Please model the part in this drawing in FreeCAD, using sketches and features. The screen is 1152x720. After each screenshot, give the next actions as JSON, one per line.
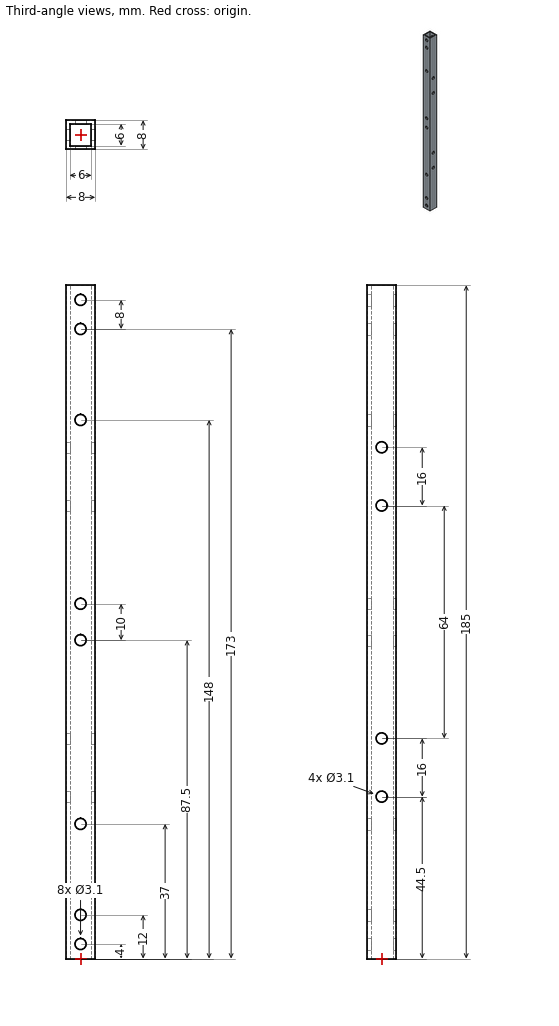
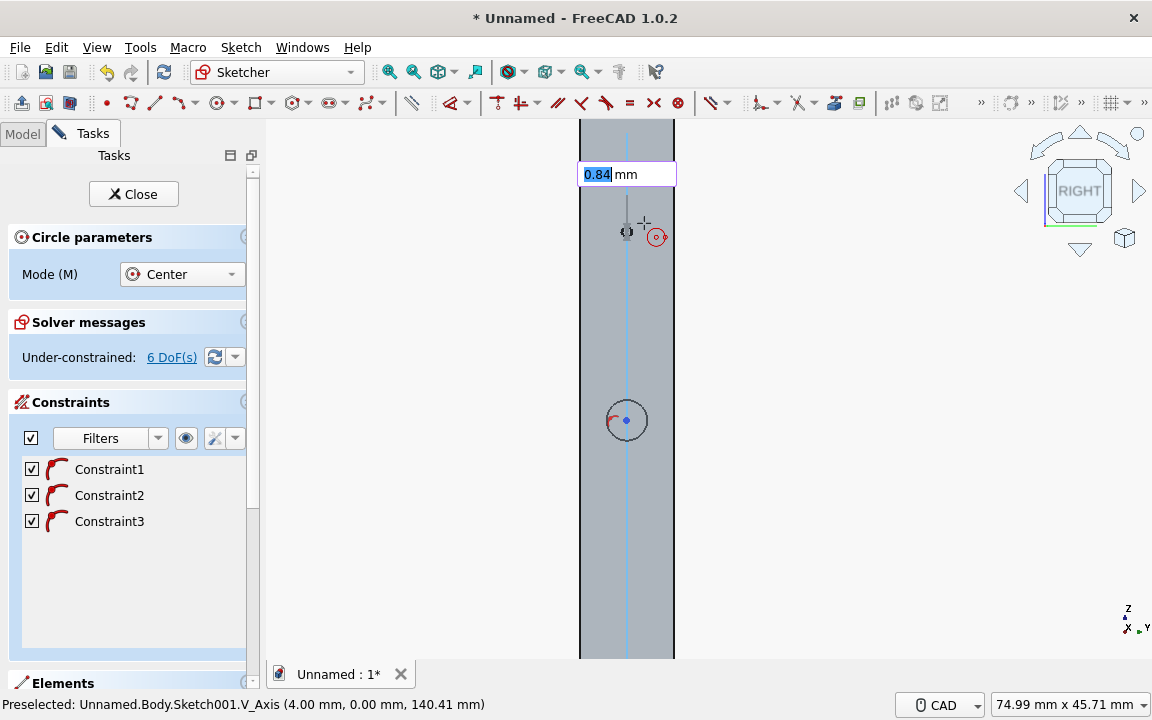
{"action": "left_click", "coordinate": [644, 220]}
{"action": "key", "text": "Escape"}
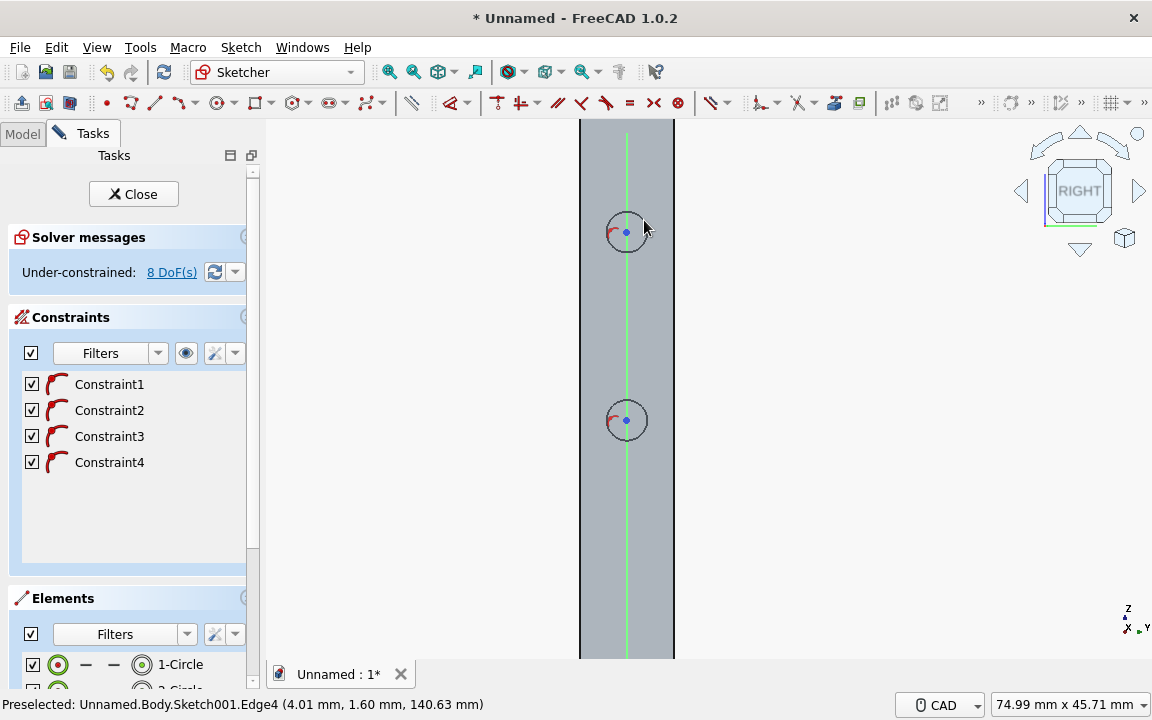
{"action": "scroll", "coordinate": [644, 223], "scroll_direction": "down", "scroll_amount": 8}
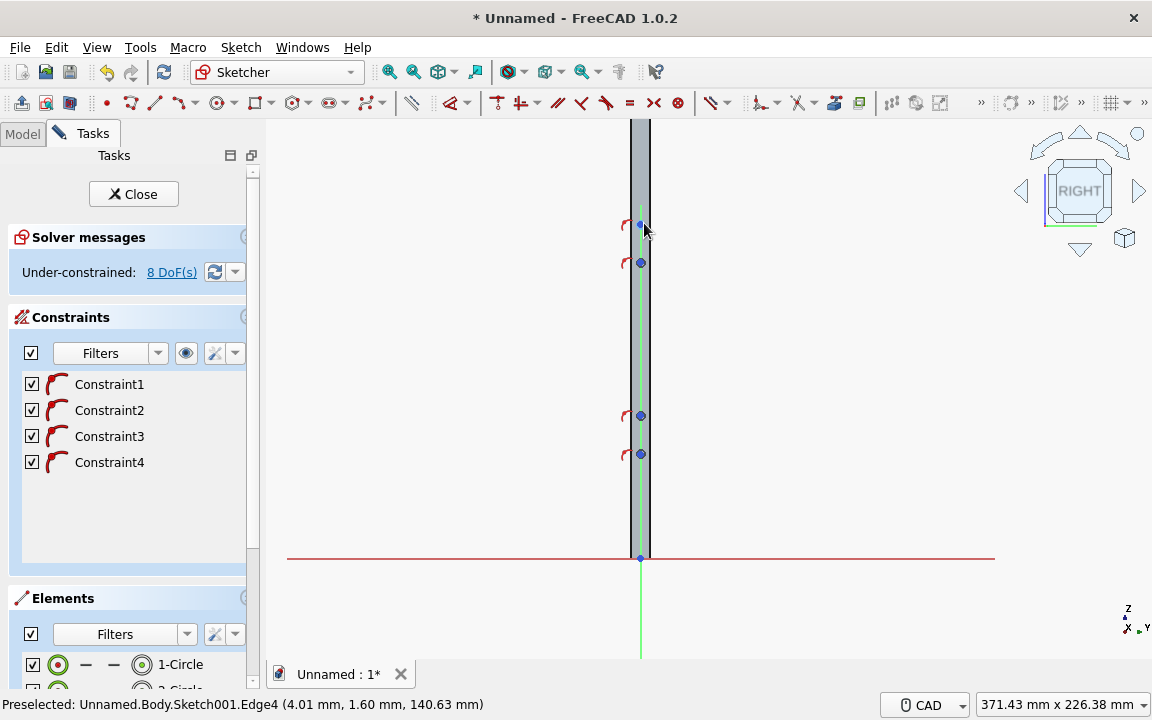
{"action": "scroll", "coordinate": [644, 451], "scroll_direction": "up", "scroll_amount": 8}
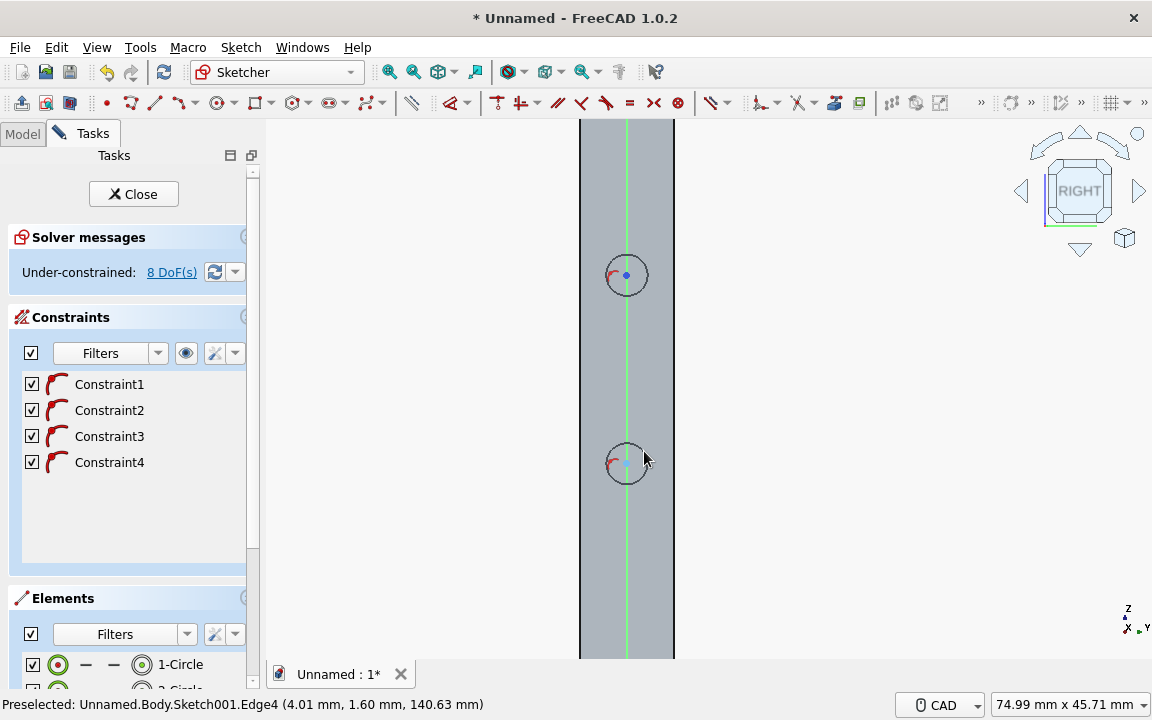
{"action": "left_click", "coordinate": [641, 449]}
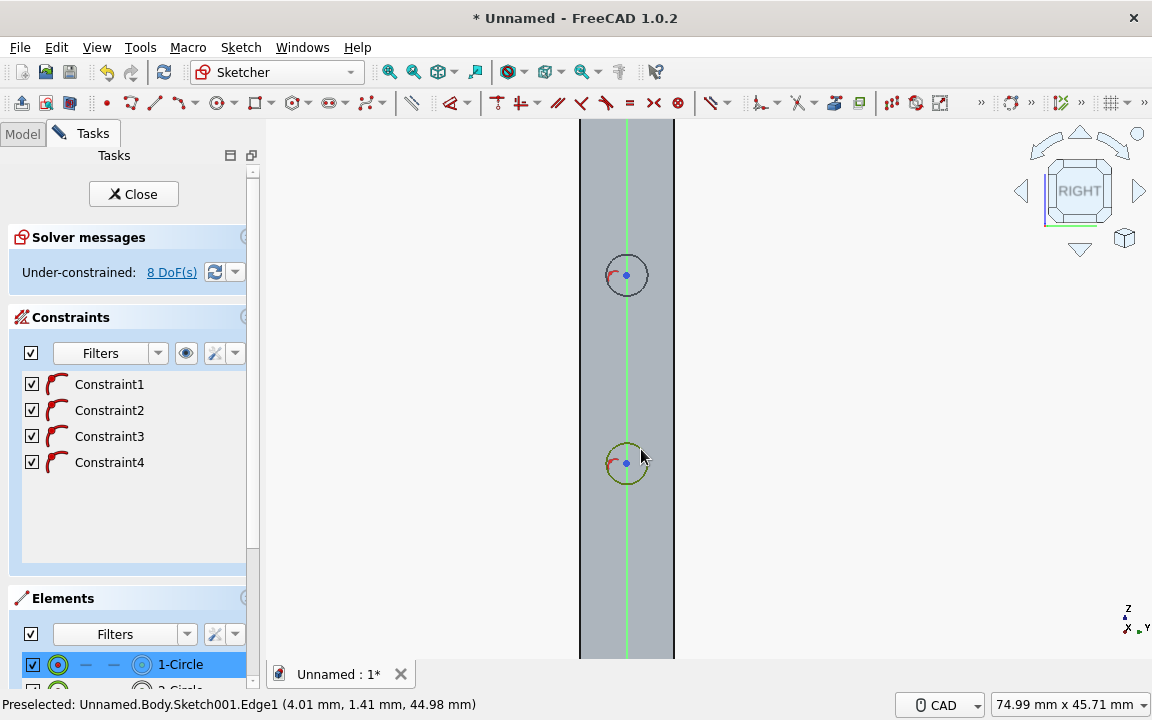
{"action": "left_click", "coordinate": [642, 261]}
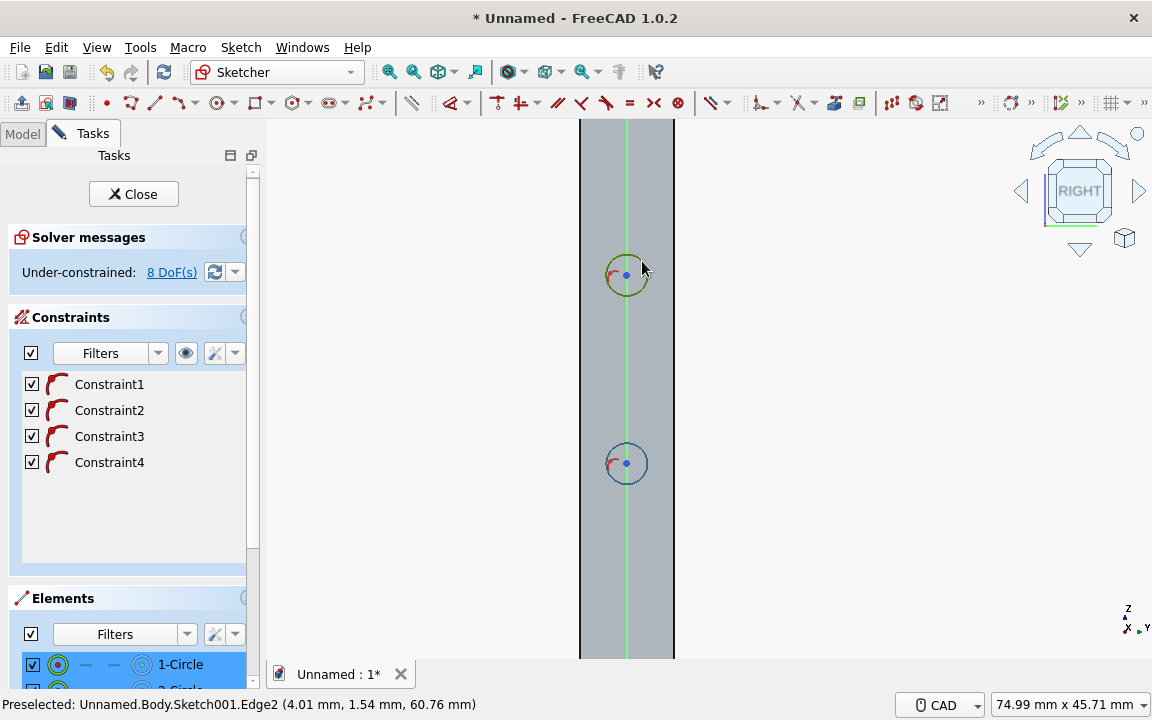
{"action": "scroll", "coordinate": [644, 451], "scroll_direction": "down", "scroll_amount": 8}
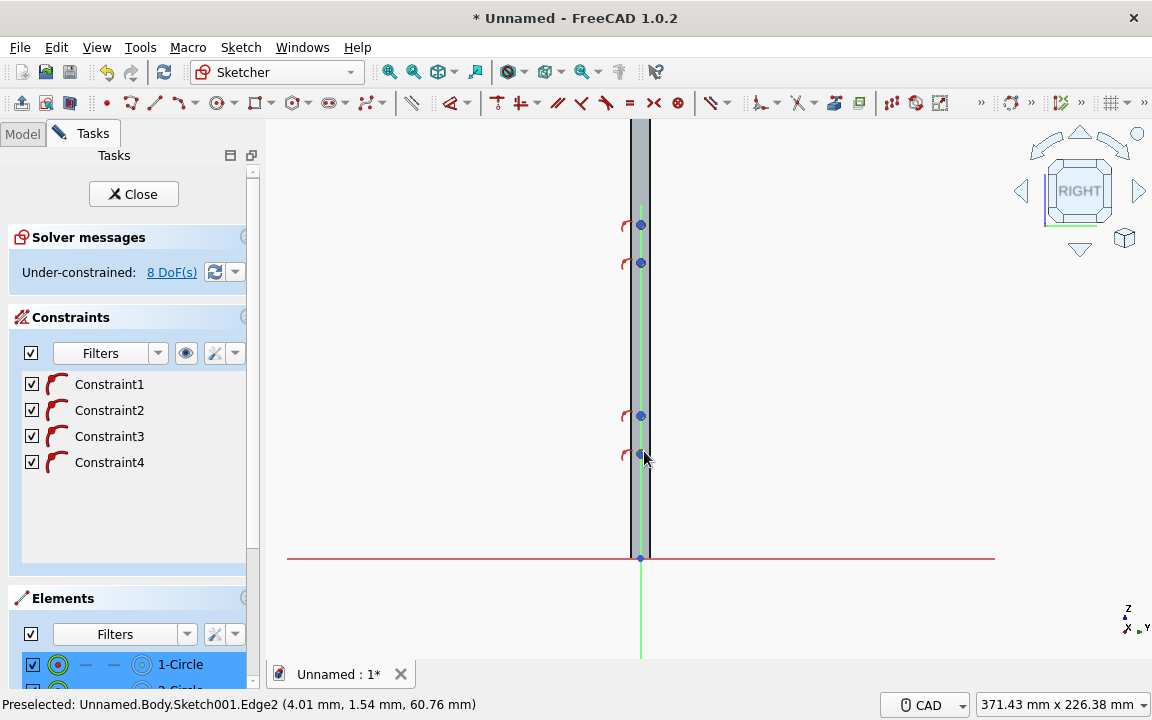
{"action": "scroll", "coordinate": [644, 260], "scroll_direction": "up", "scroll_amount": 8}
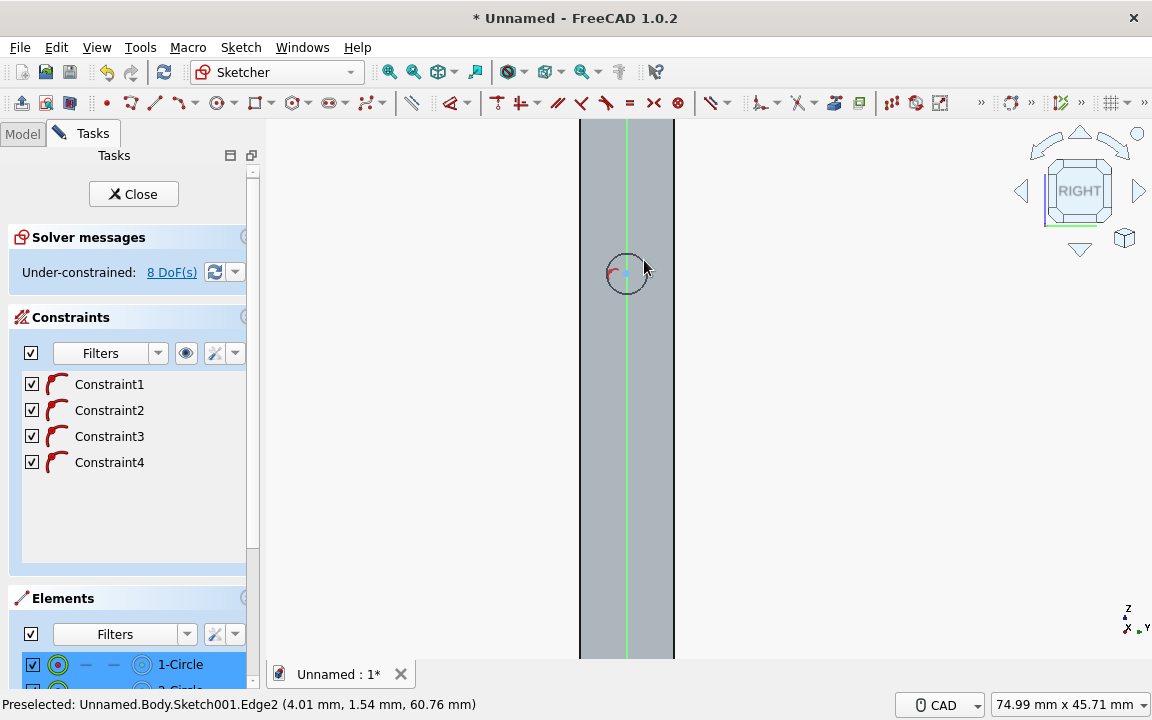
{"action": "left_click", "coordinate": [641, 259]}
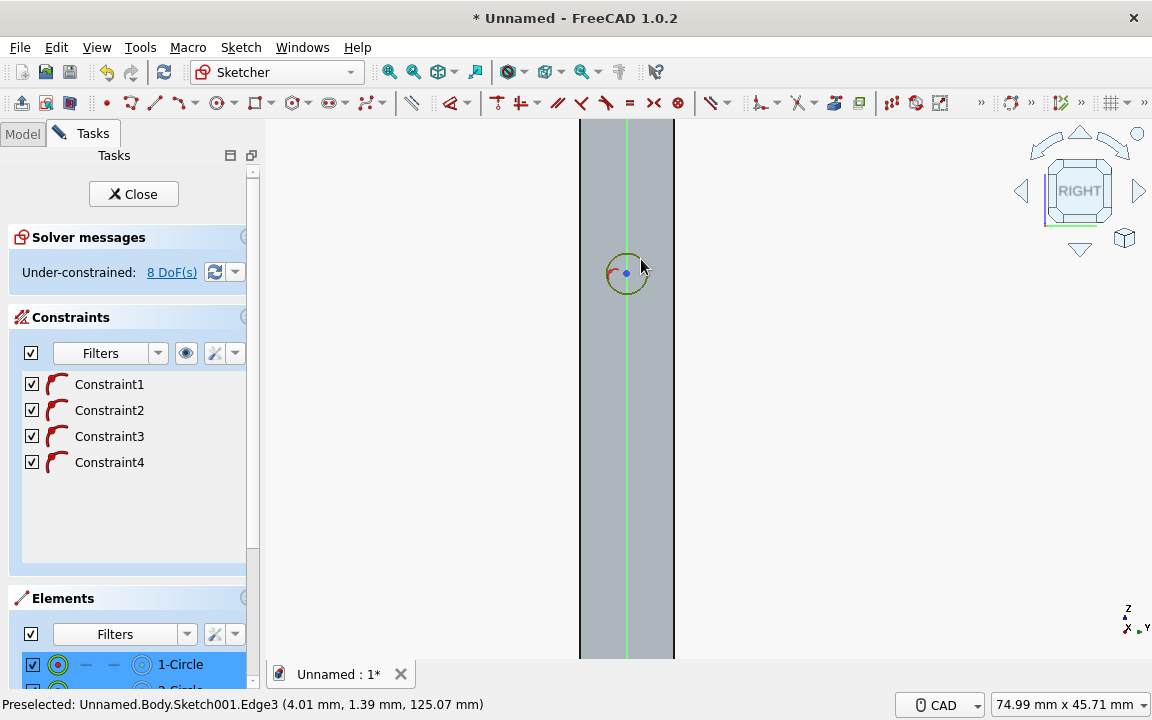
{"action": "scroll", "coordinate": [644, 260], "scroll_direction": "down", "scroll_amount": 8}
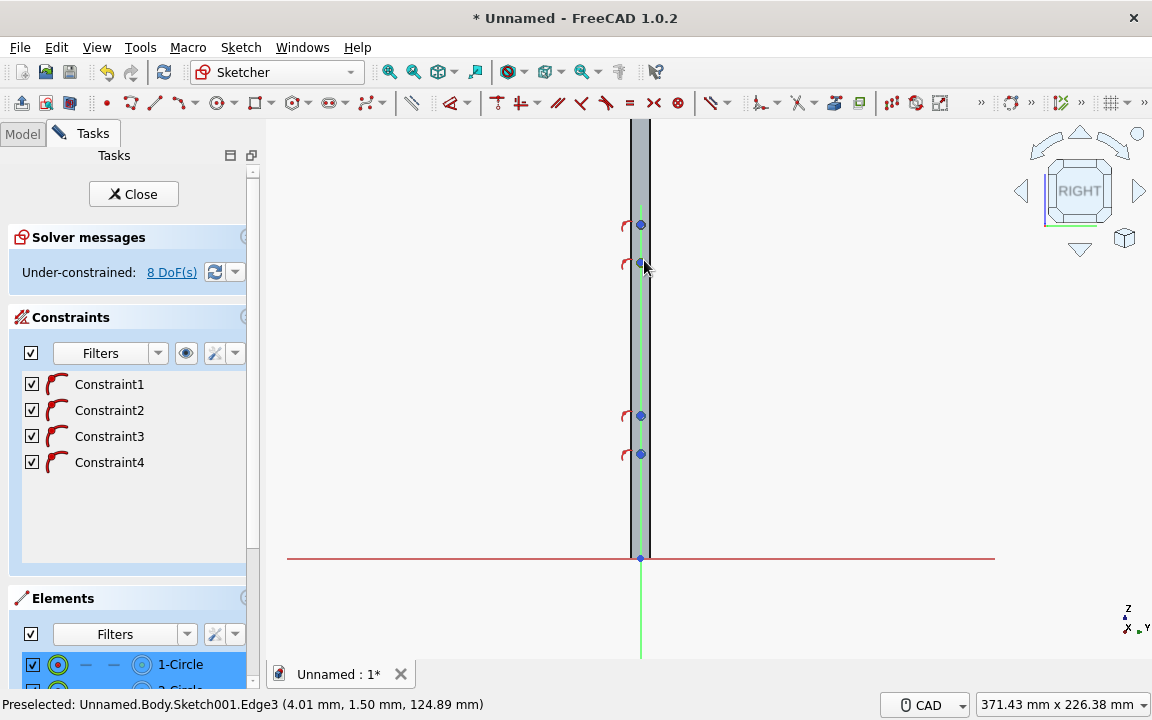
{"action": "scroll", "coordinate": [644, 222], "scroll_direction": "up", "scroll_amount": 8}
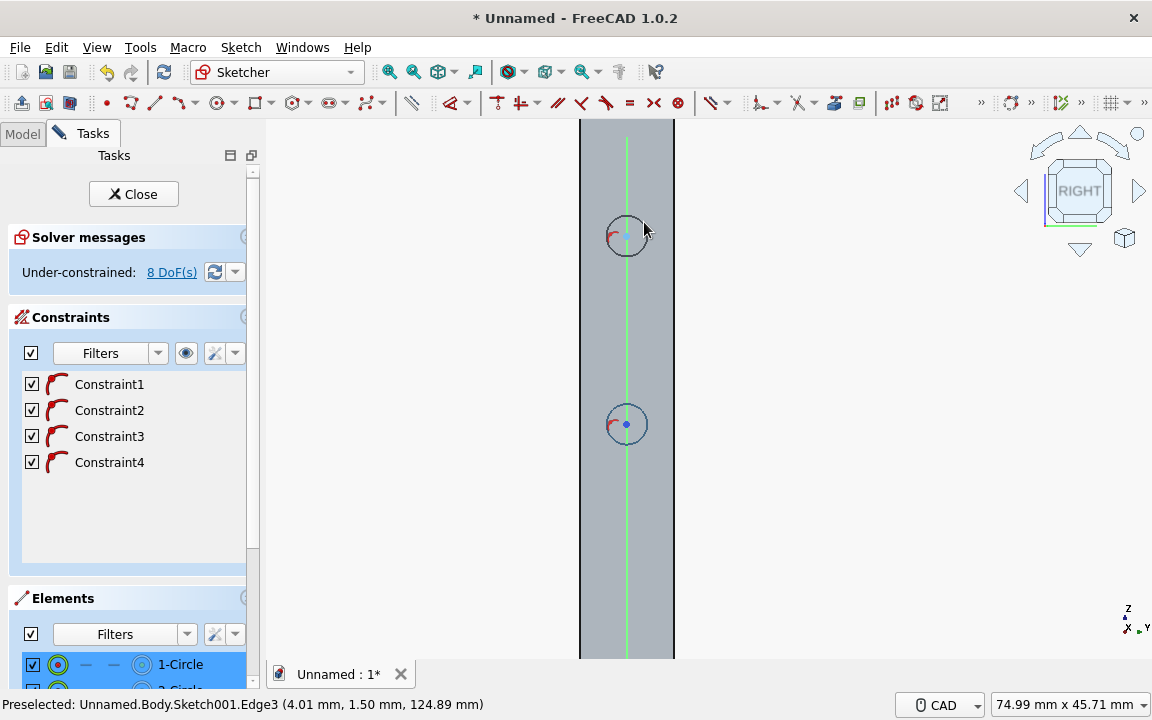
{"action": "left_click", "coordinate": [641, 222]}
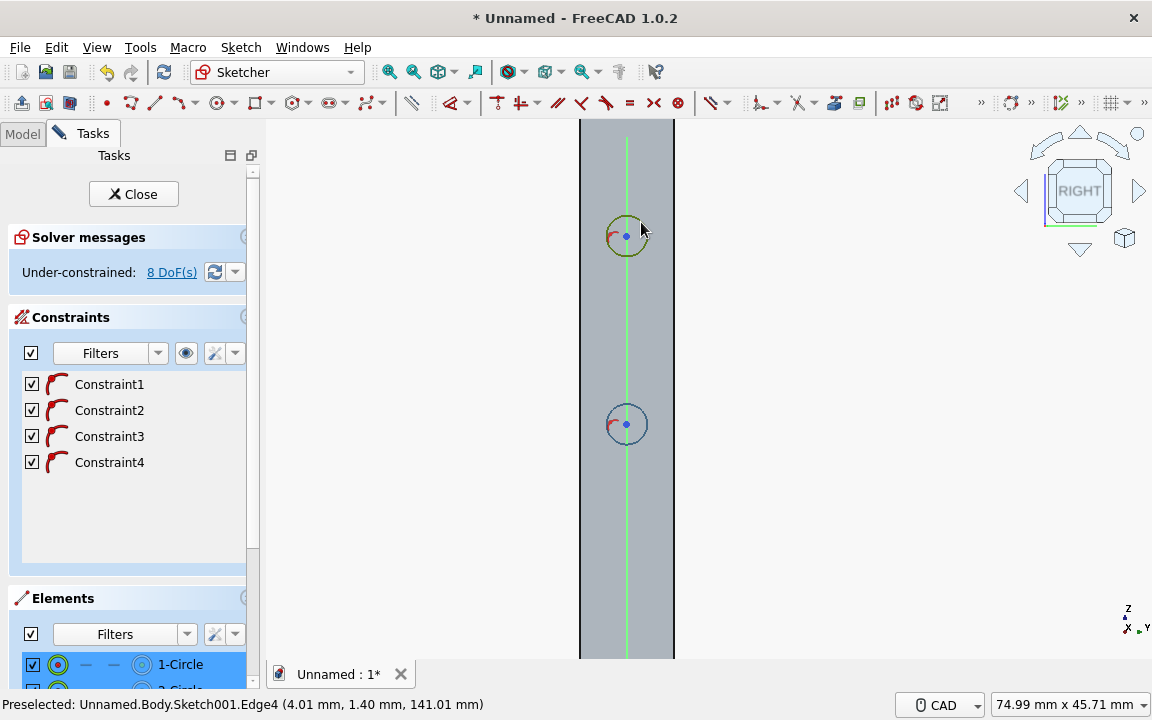
{"action": "left_click", "coordinate": [630, 104]}